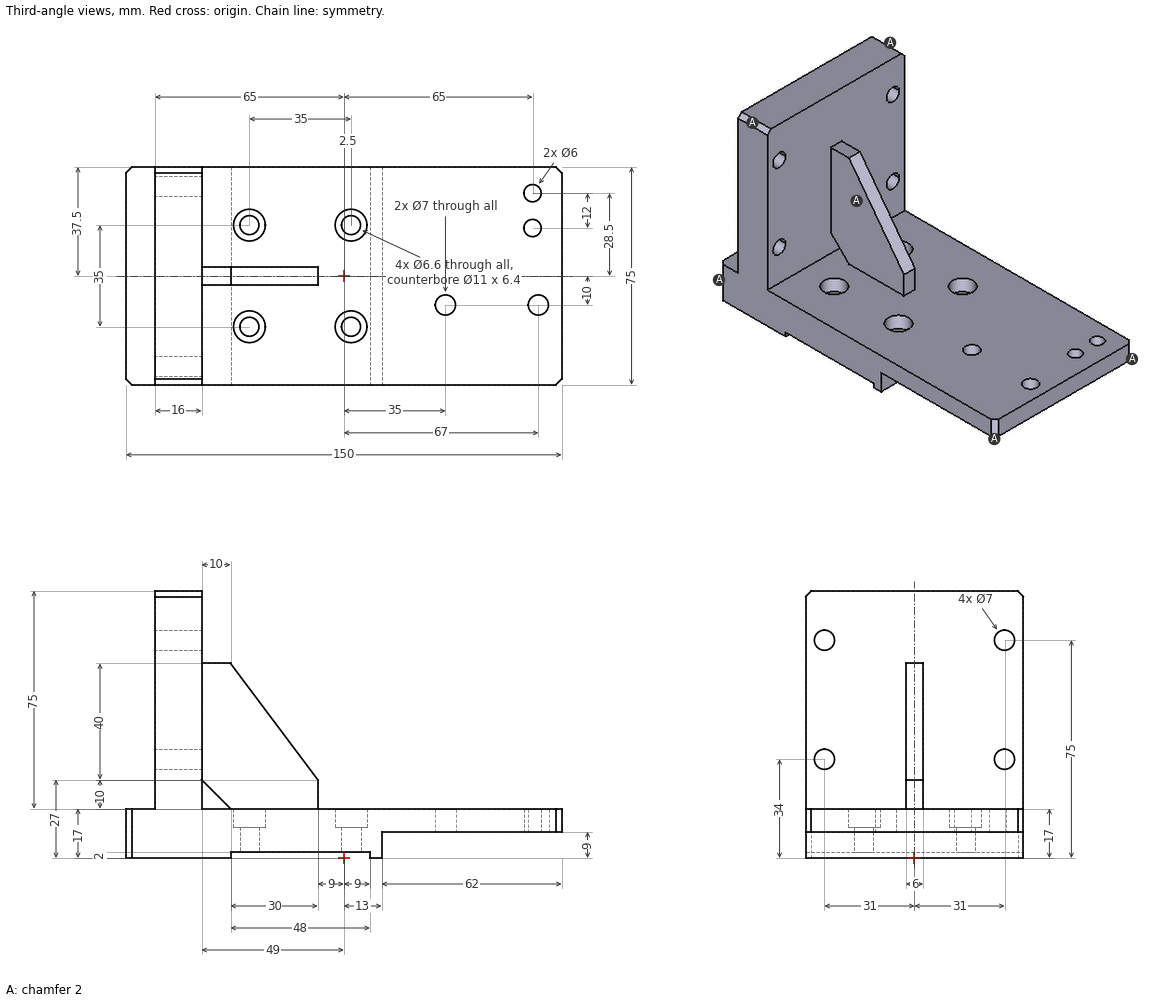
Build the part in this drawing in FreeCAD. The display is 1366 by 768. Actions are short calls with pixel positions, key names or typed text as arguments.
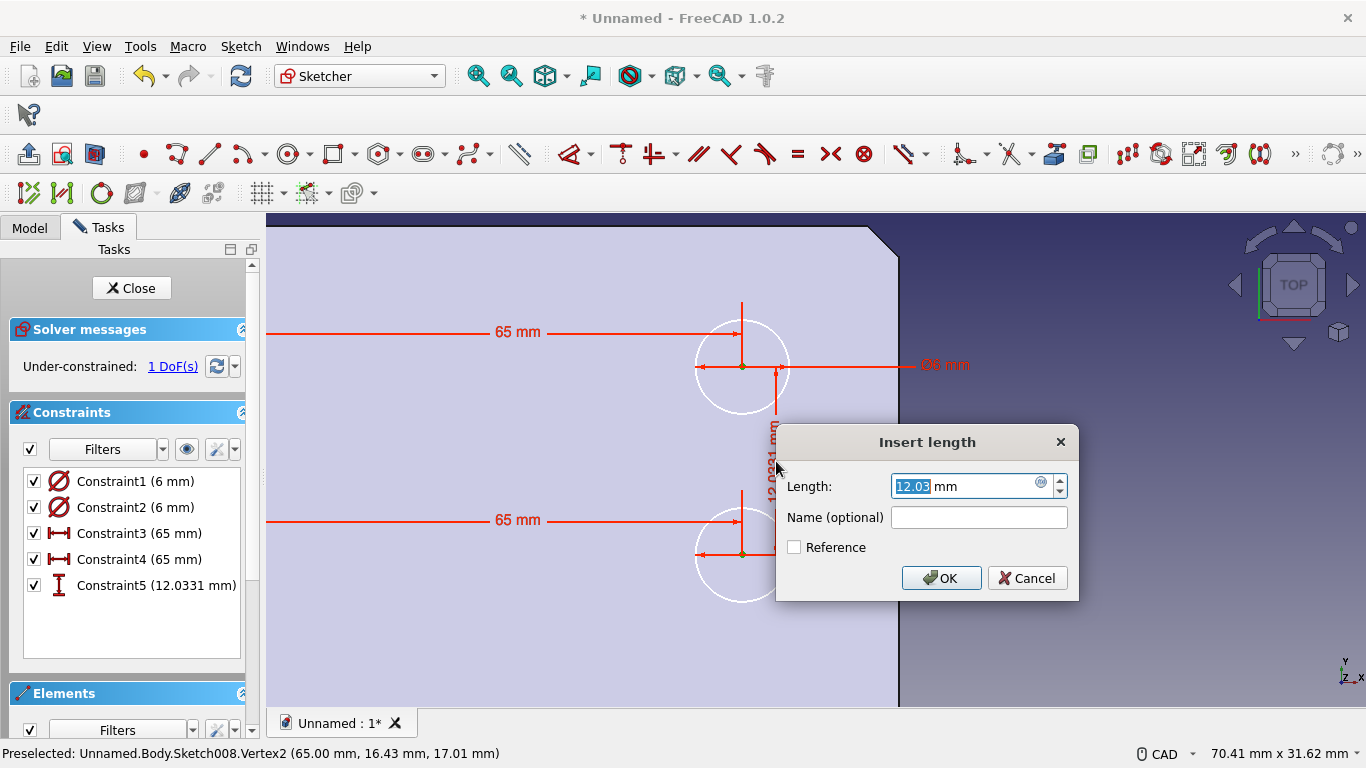
text(12)
key(Return)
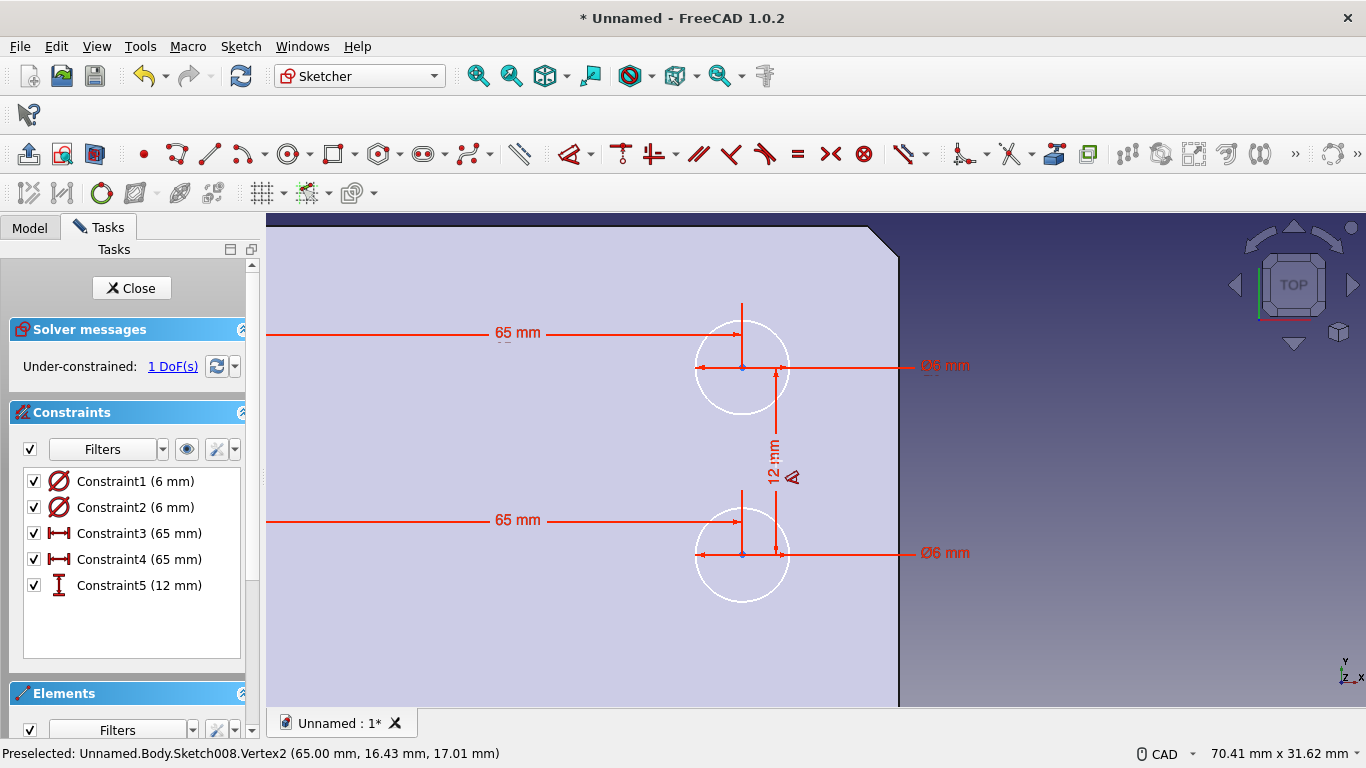
click(742, 368)
click(776, 632)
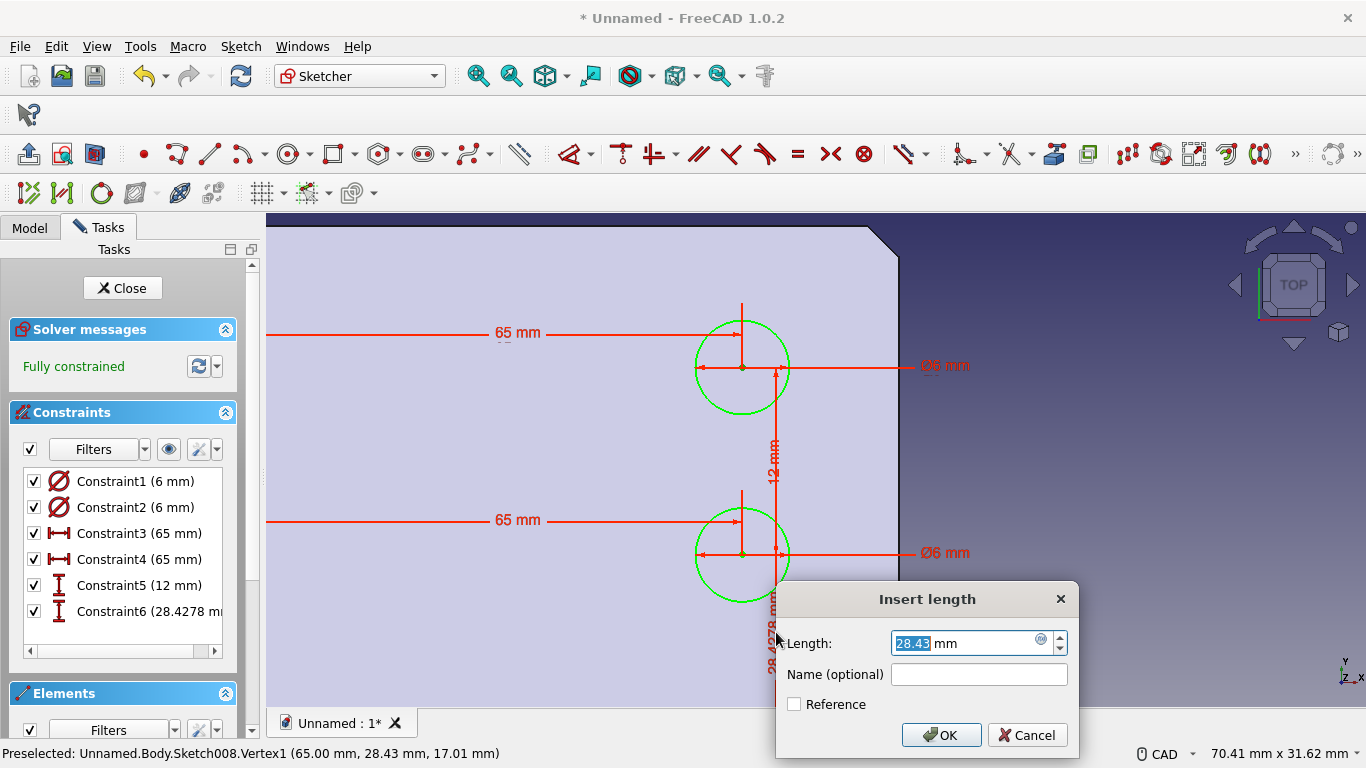
text(28.5)
key(Return)
key(Escape)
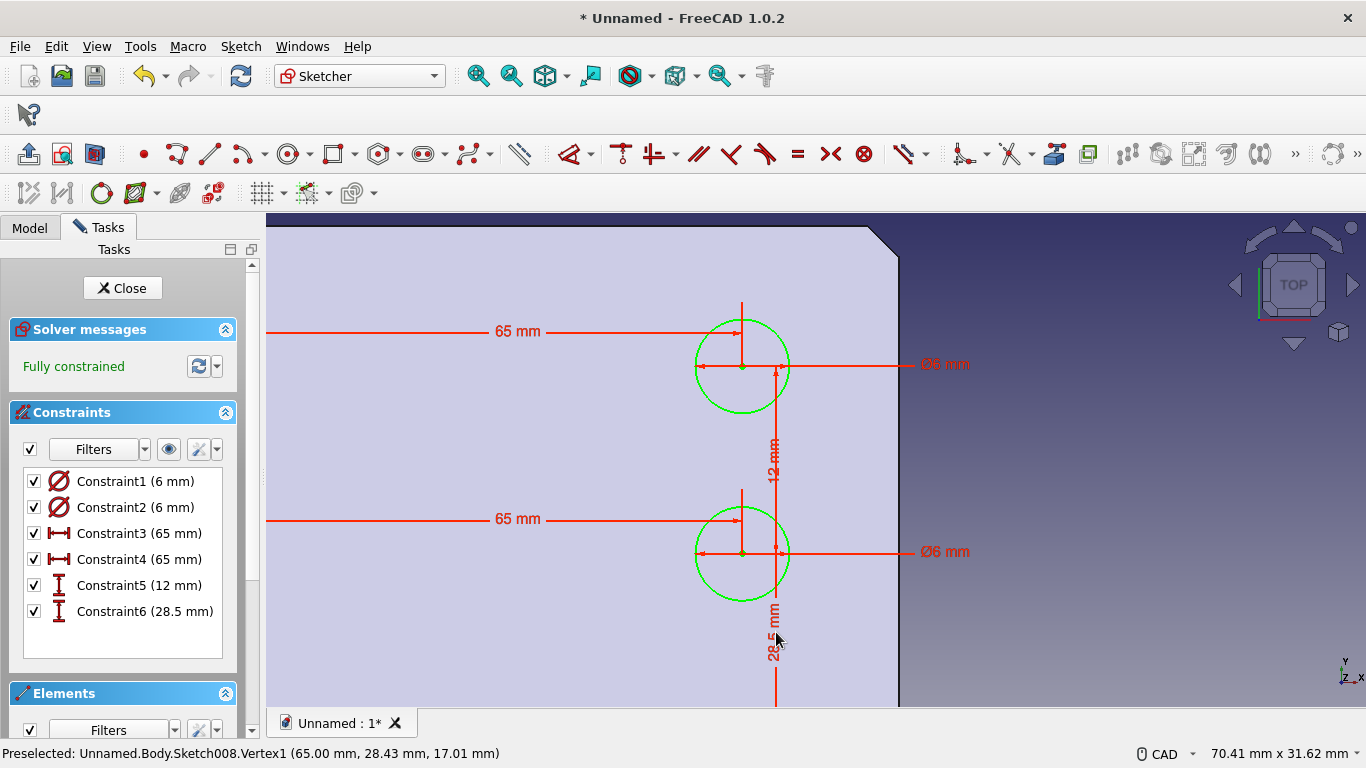
click(123, 288)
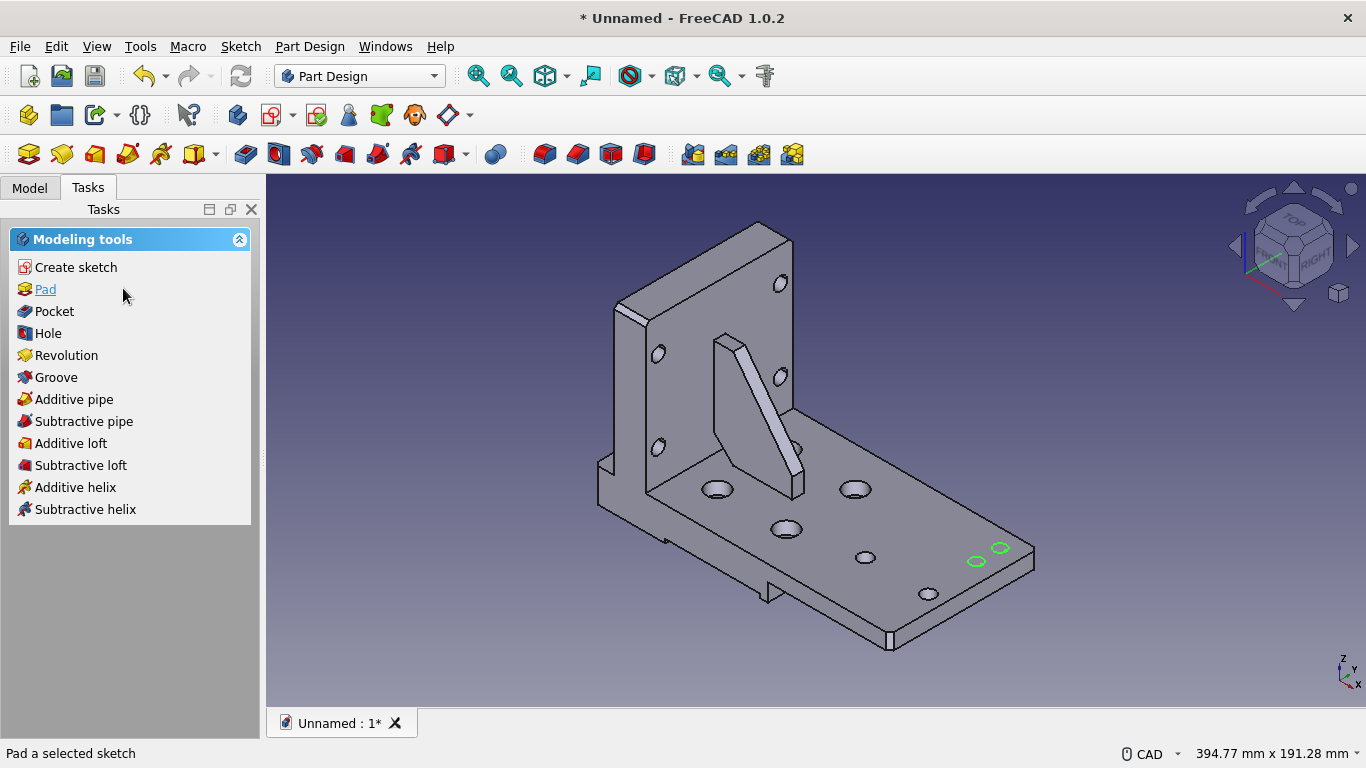
click(246, 154)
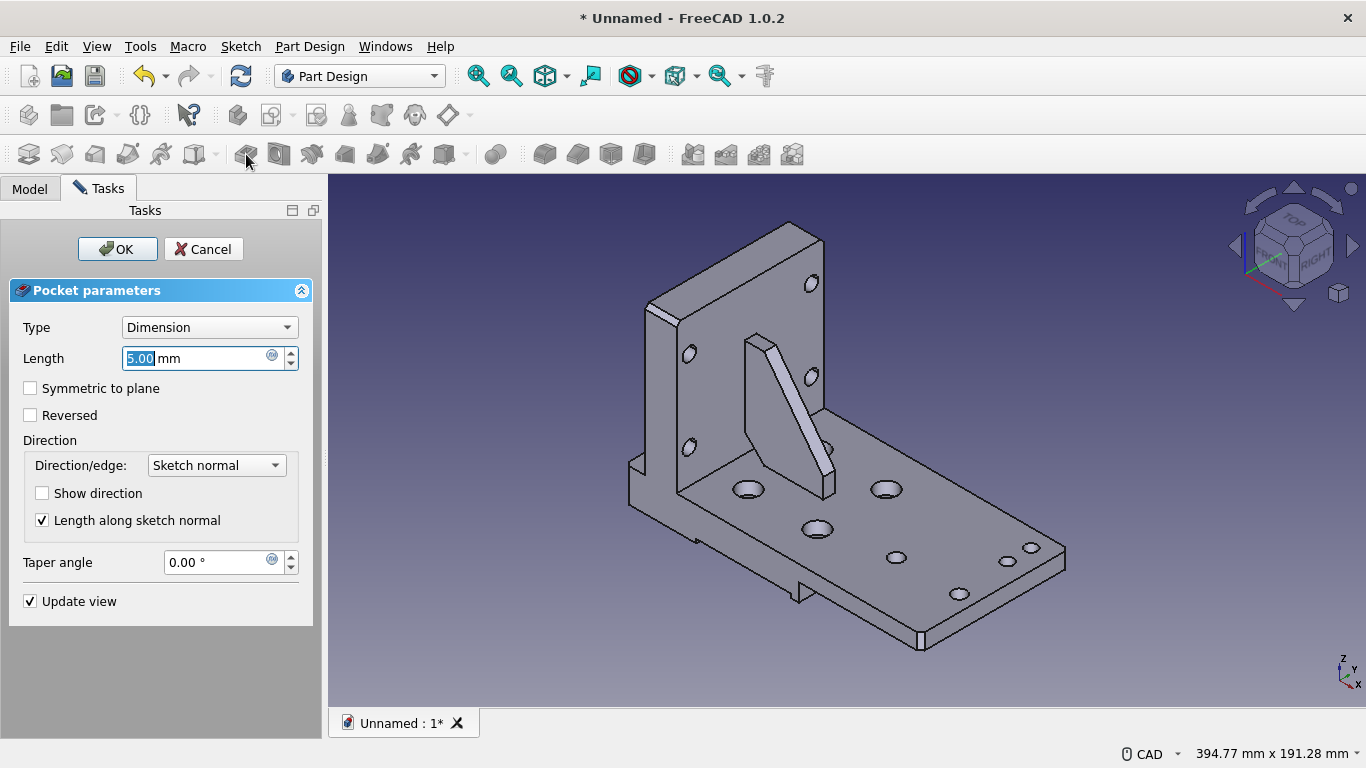
click(210, 328)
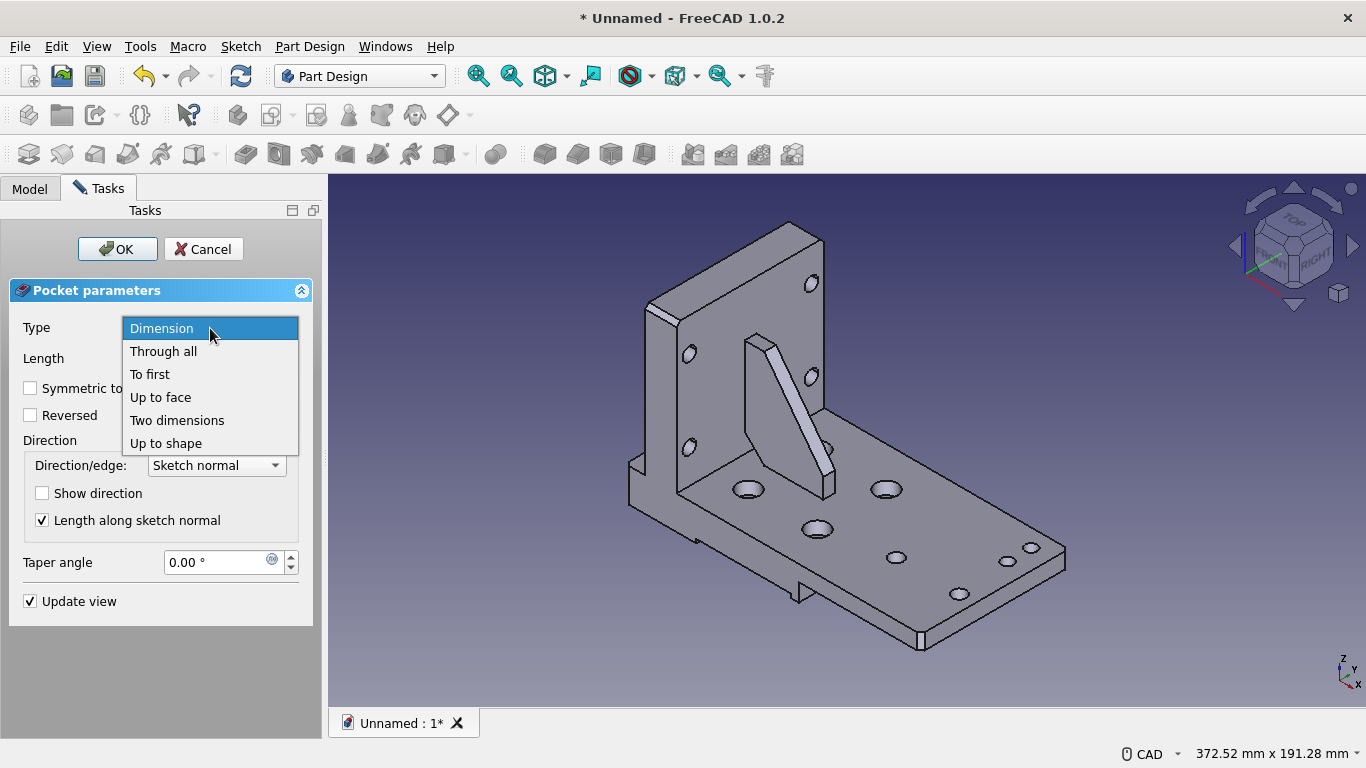
click(208, 352)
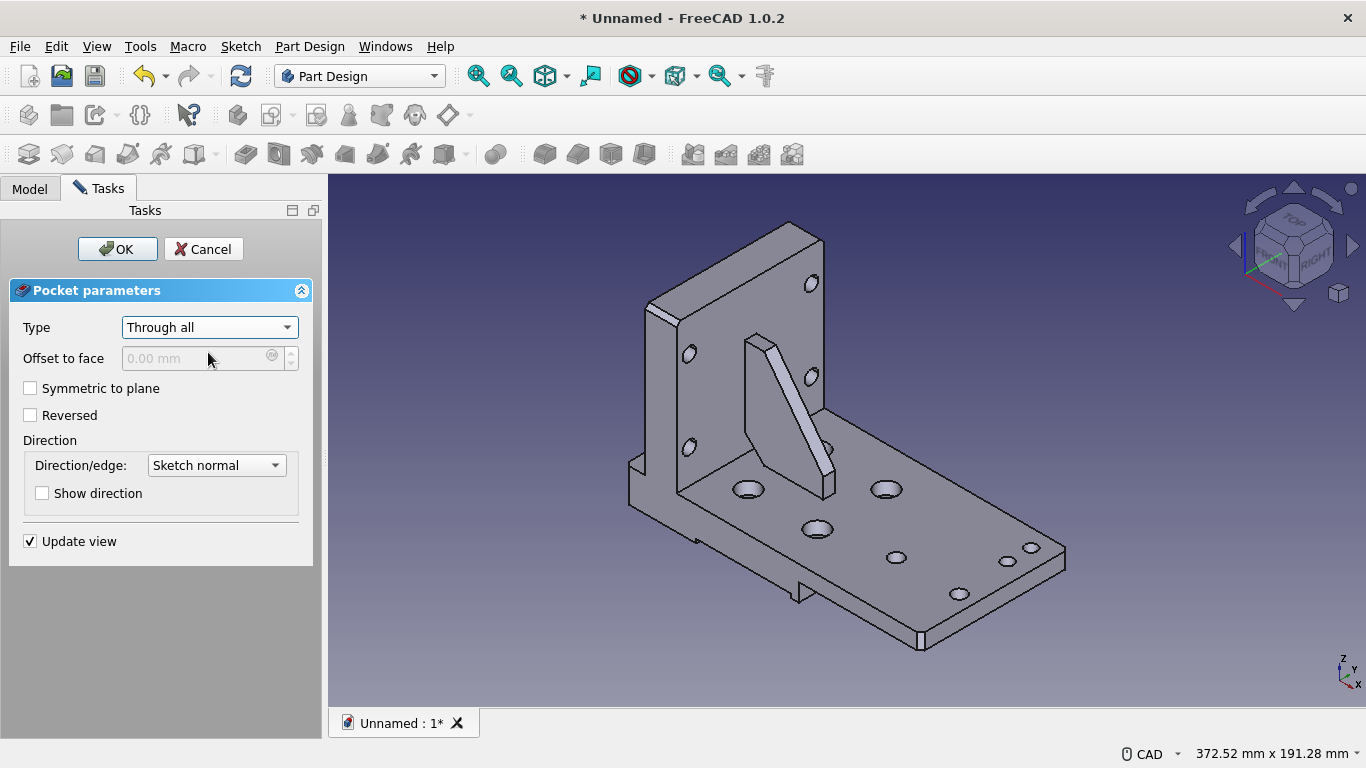
click(118, 249)